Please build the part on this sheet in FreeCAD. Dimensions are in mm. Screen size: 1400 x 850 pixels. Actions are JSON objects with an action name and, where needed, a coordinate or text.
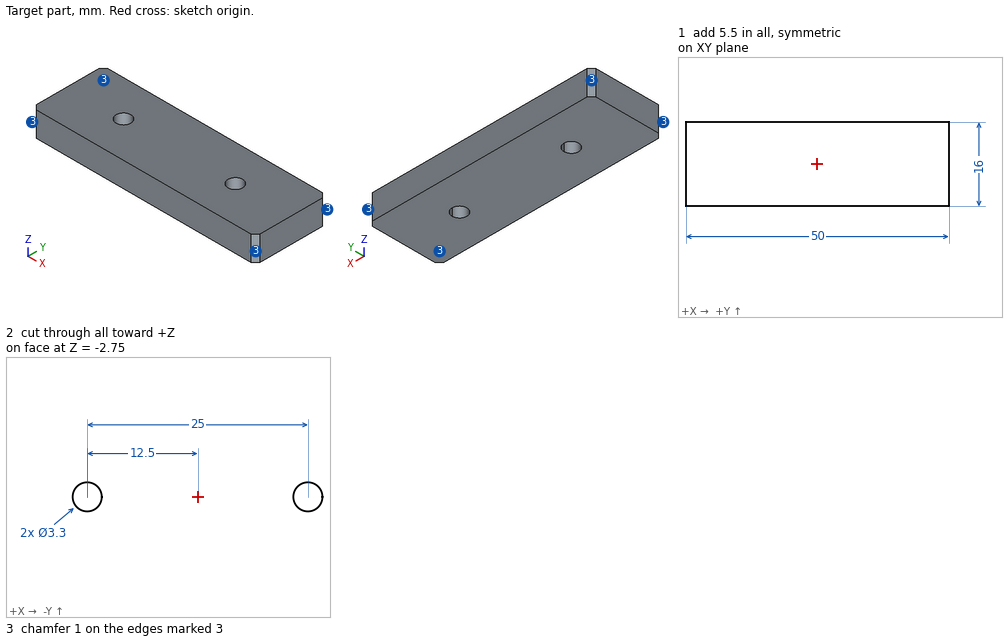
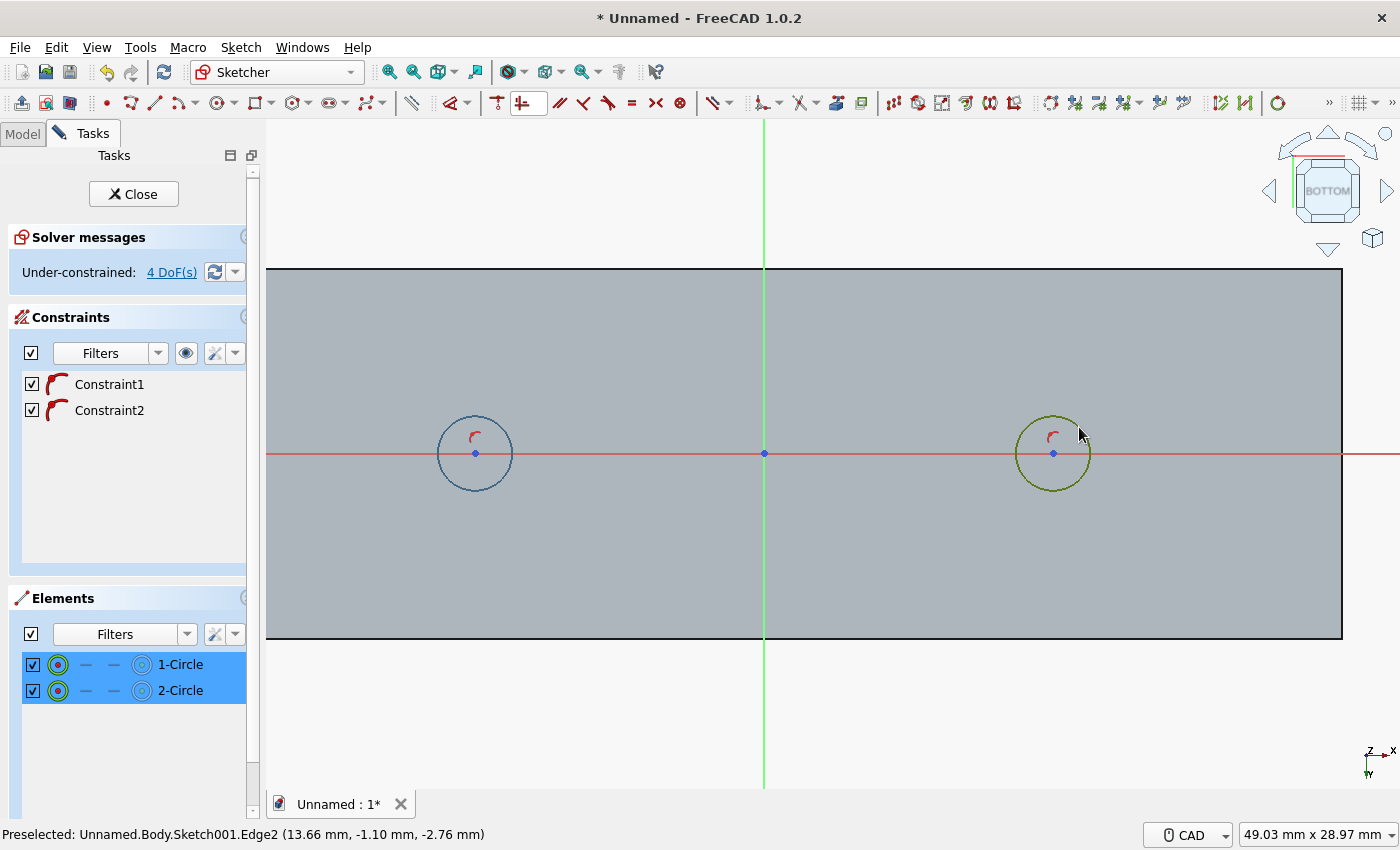
{"action": "left_click", "coordinate": [632, 104]}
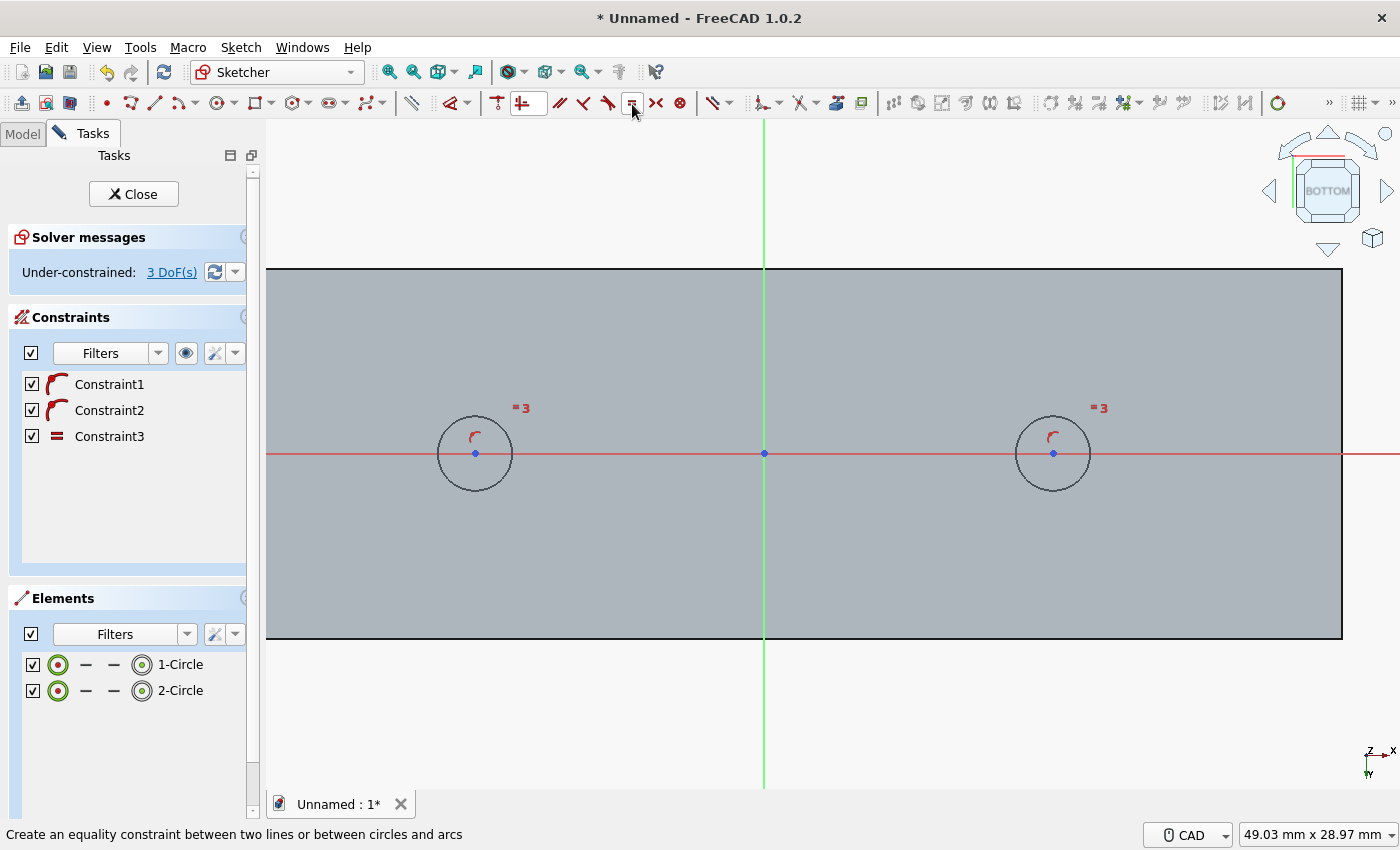
{"action": "key", "text": "d"}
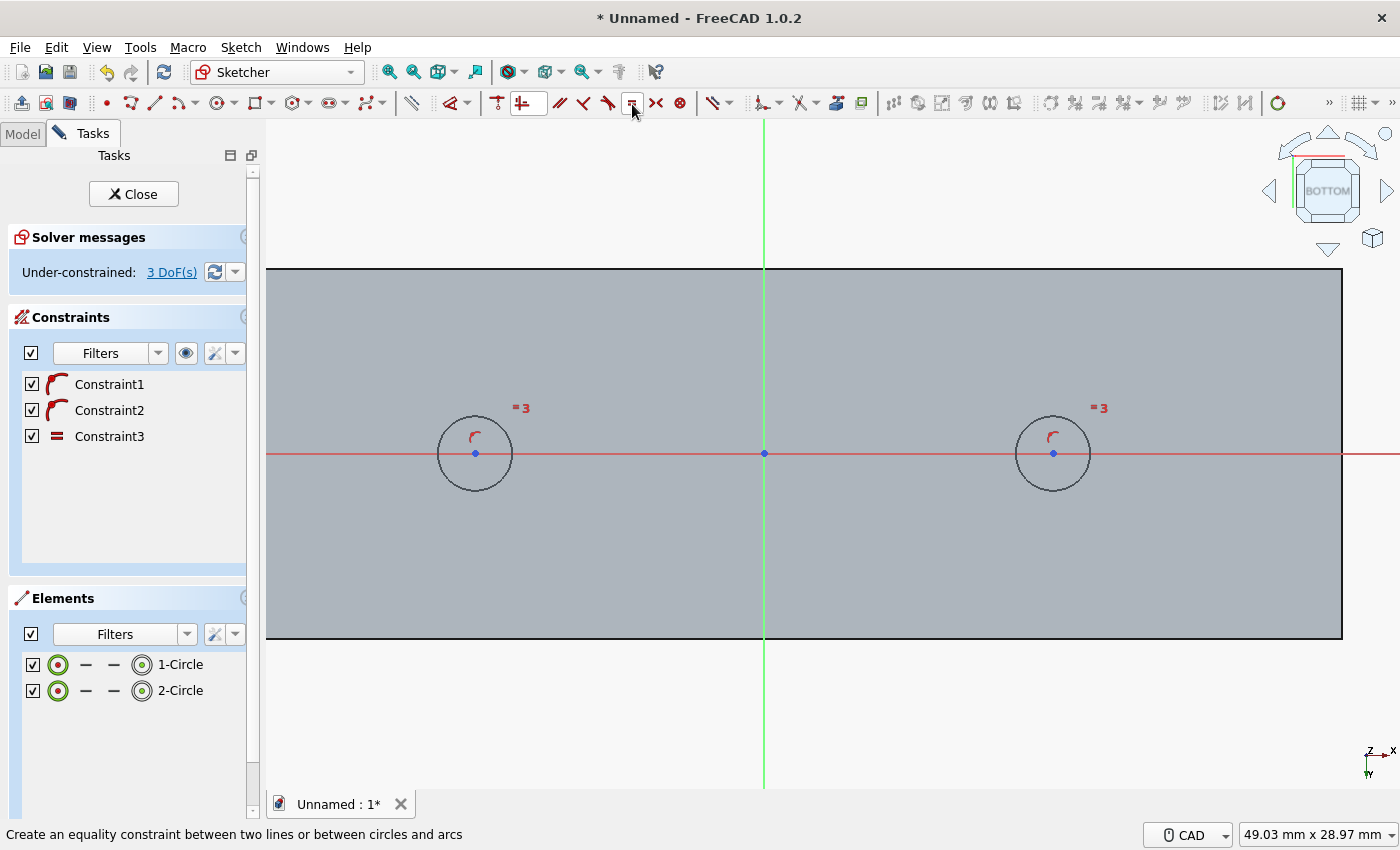
{"action": "left_click", "coordinate": [501, 427]}
{"action": "left_click", "coordinate": [523, 404]}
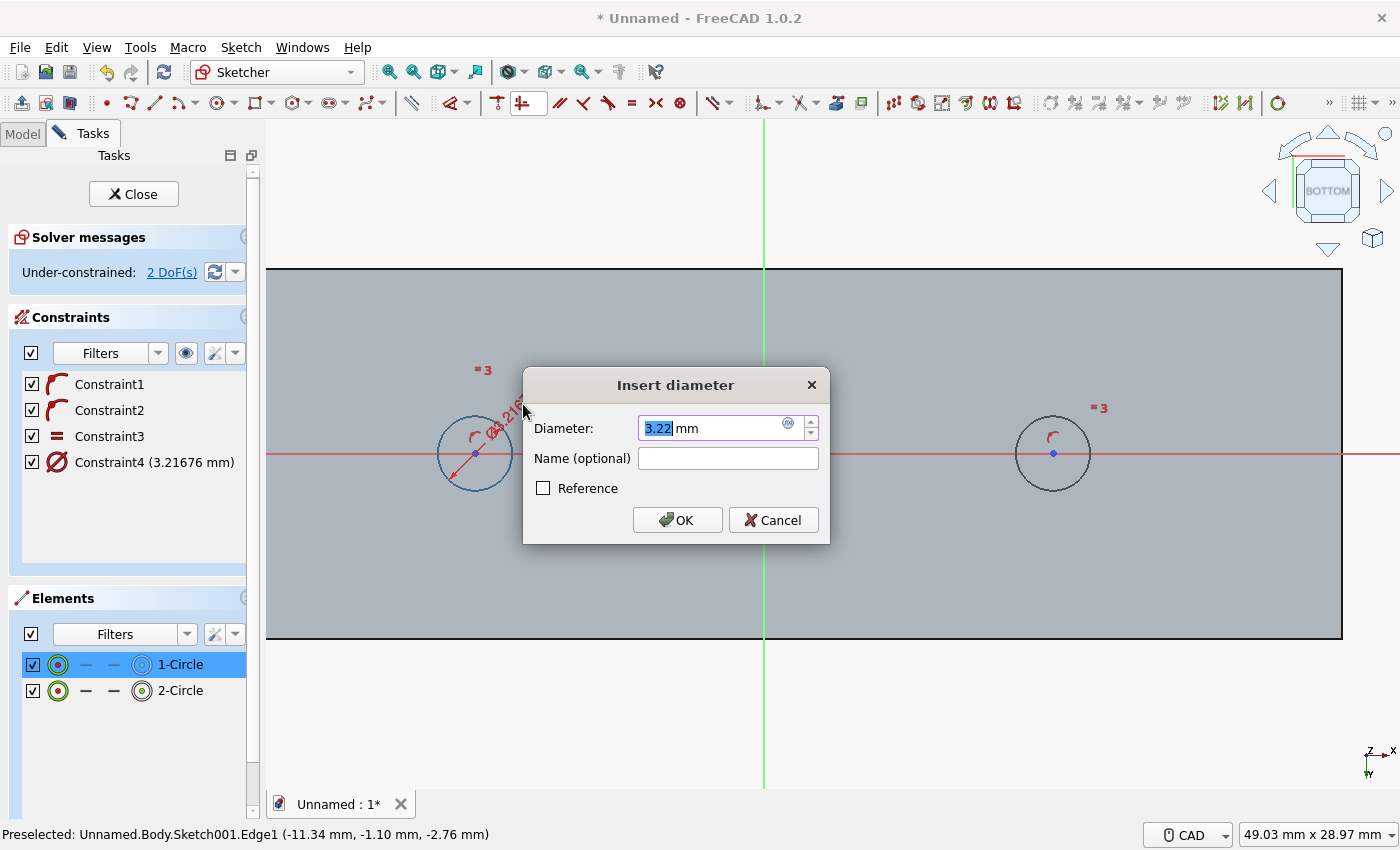
{"action": "type", "text": "3.3"}
{"action": "key", "text": "Return"}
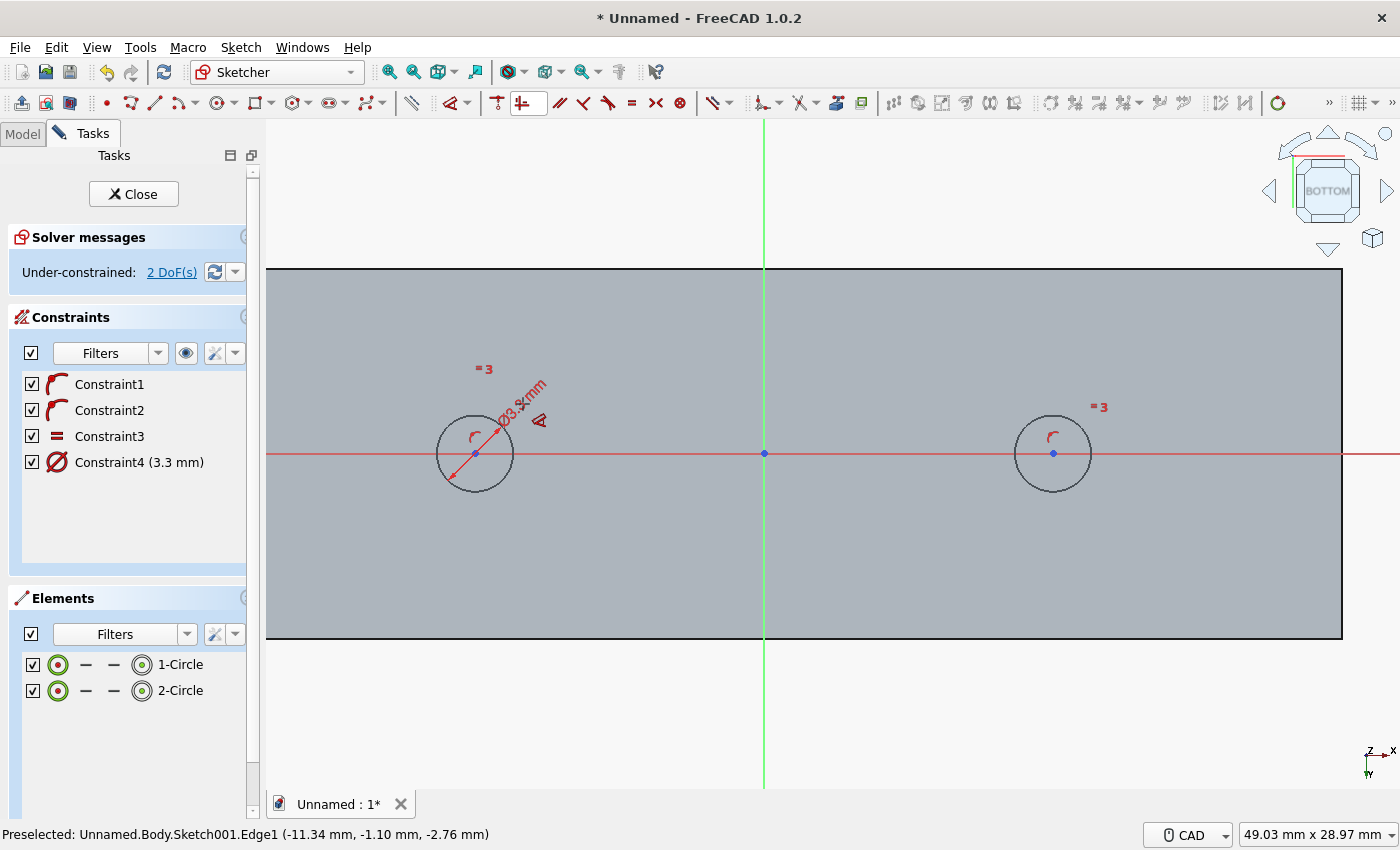
{"action": "left_click", "coordinate": [475, 454]}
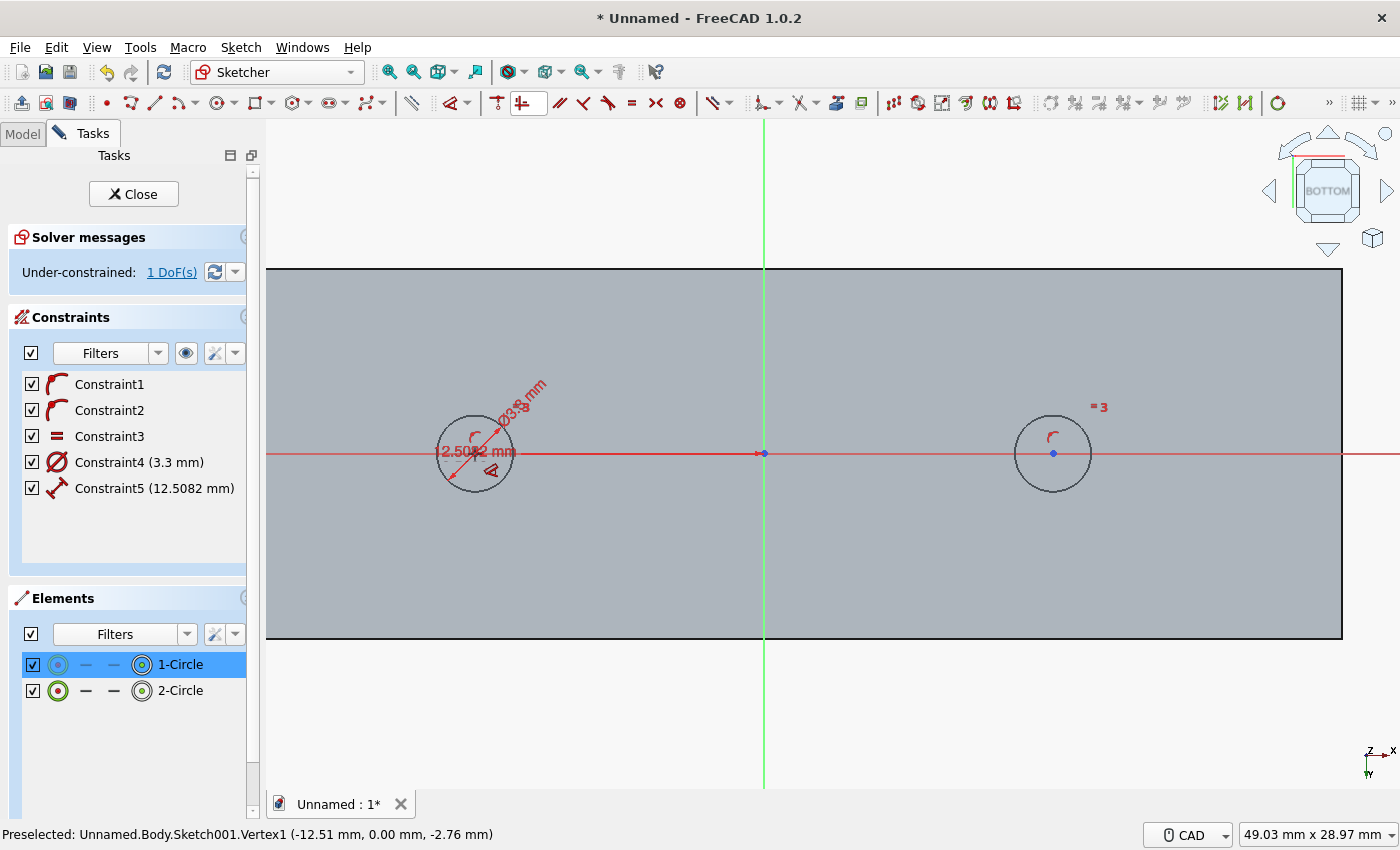
{"action": "left_click", "coordinate": [1053, 454]}
{"action": "left_click", "coordinate": [631, 488]}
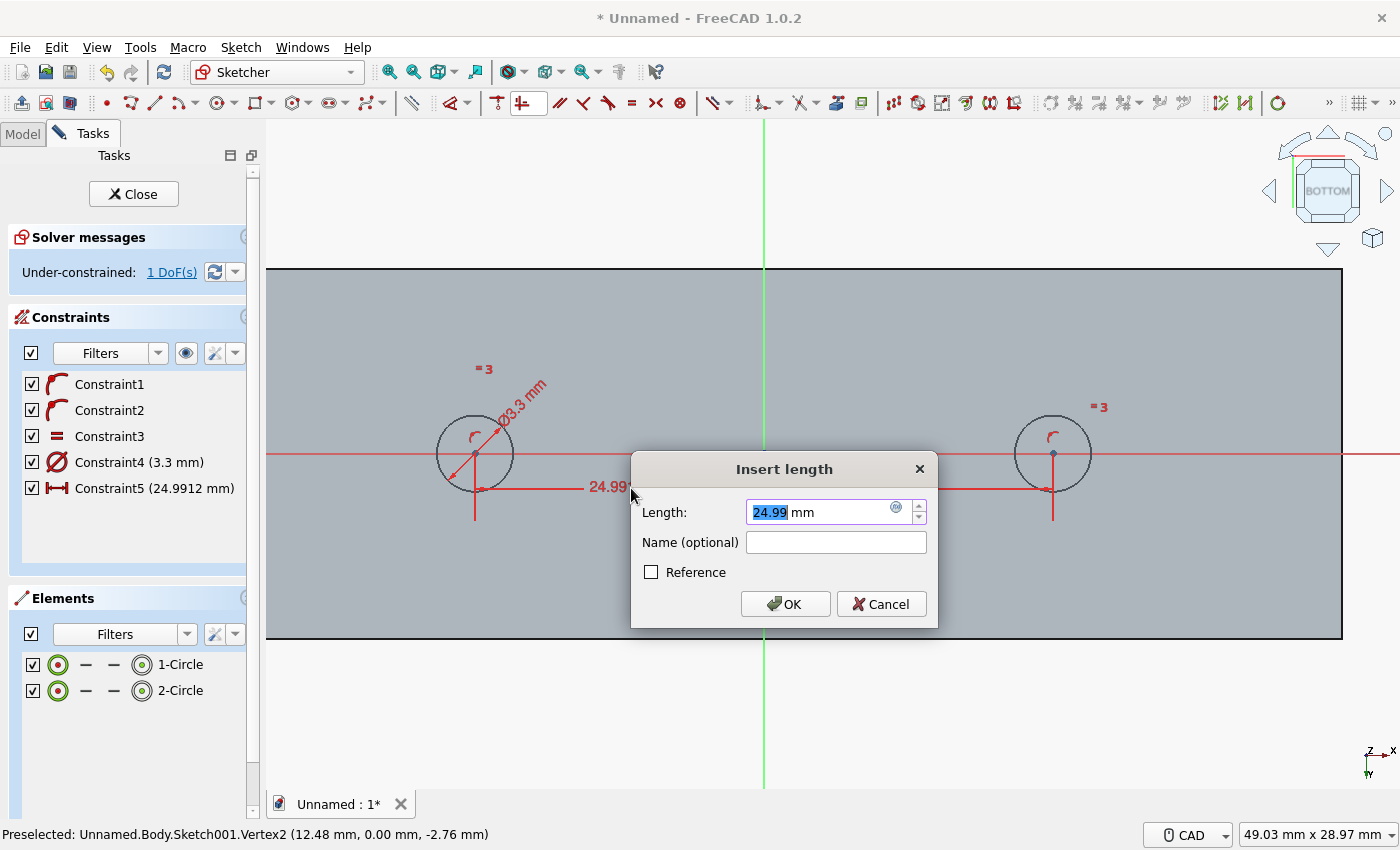
{"action": "type", "text": "25"}
{"action": "key", "text": "Return"}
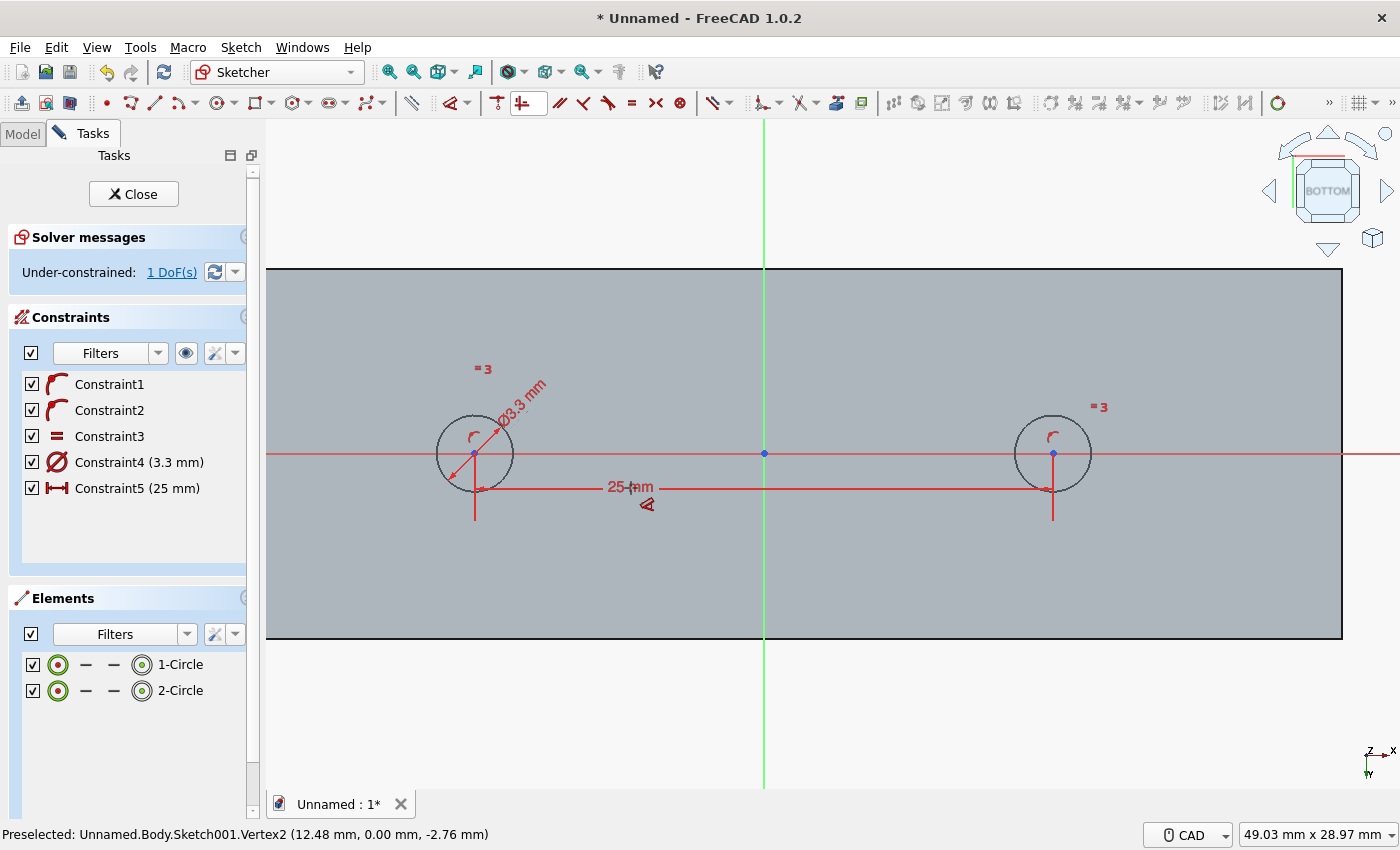
{"action": "left_click", "coordinate": [475, 454]}
{"action": "left_click", "coordinate": [553, 488]}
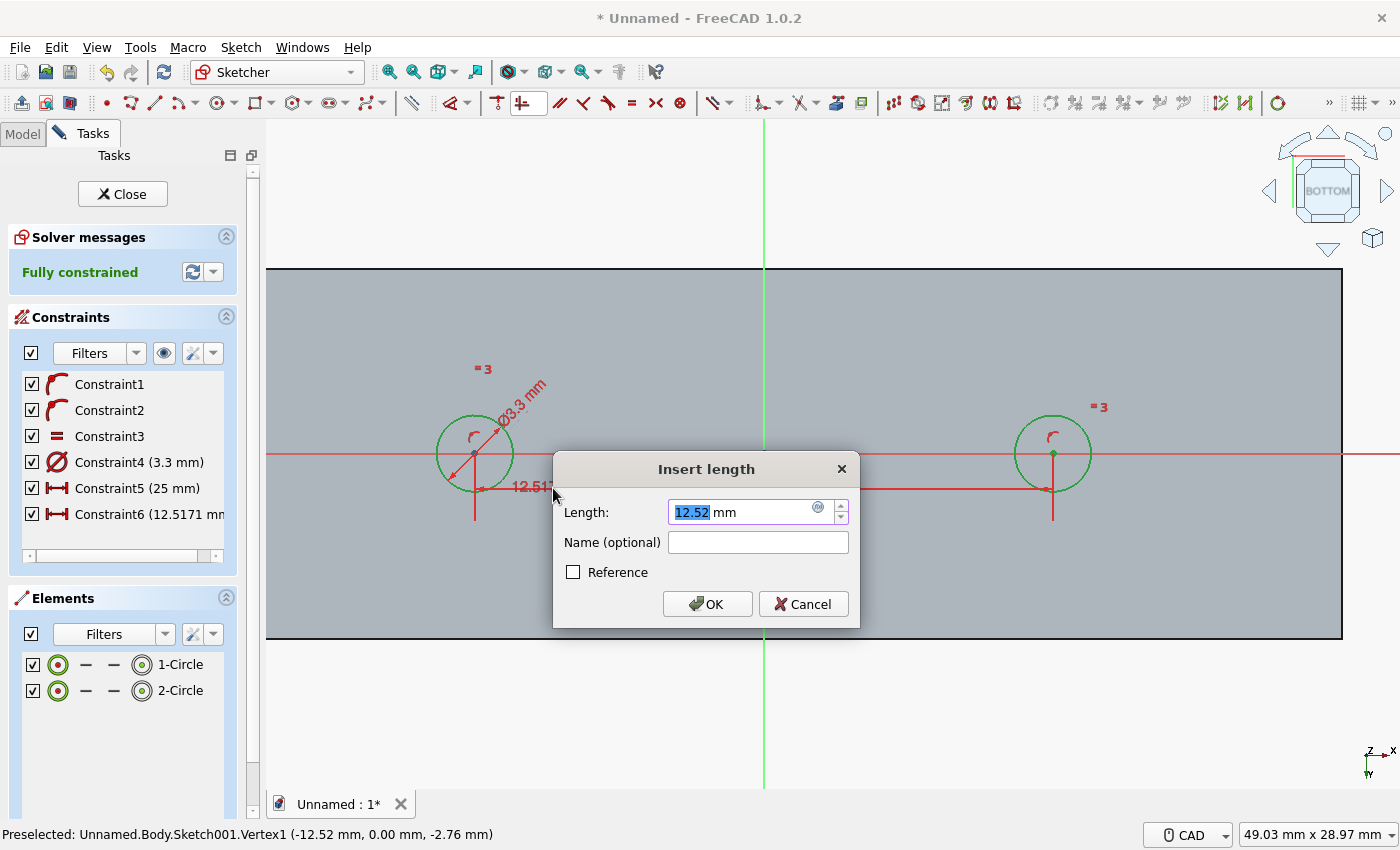
{"action": "type", "text": "12.5"}
{"action": "key", "text": "Return"}
{"action": "key", "text": "Escape"}